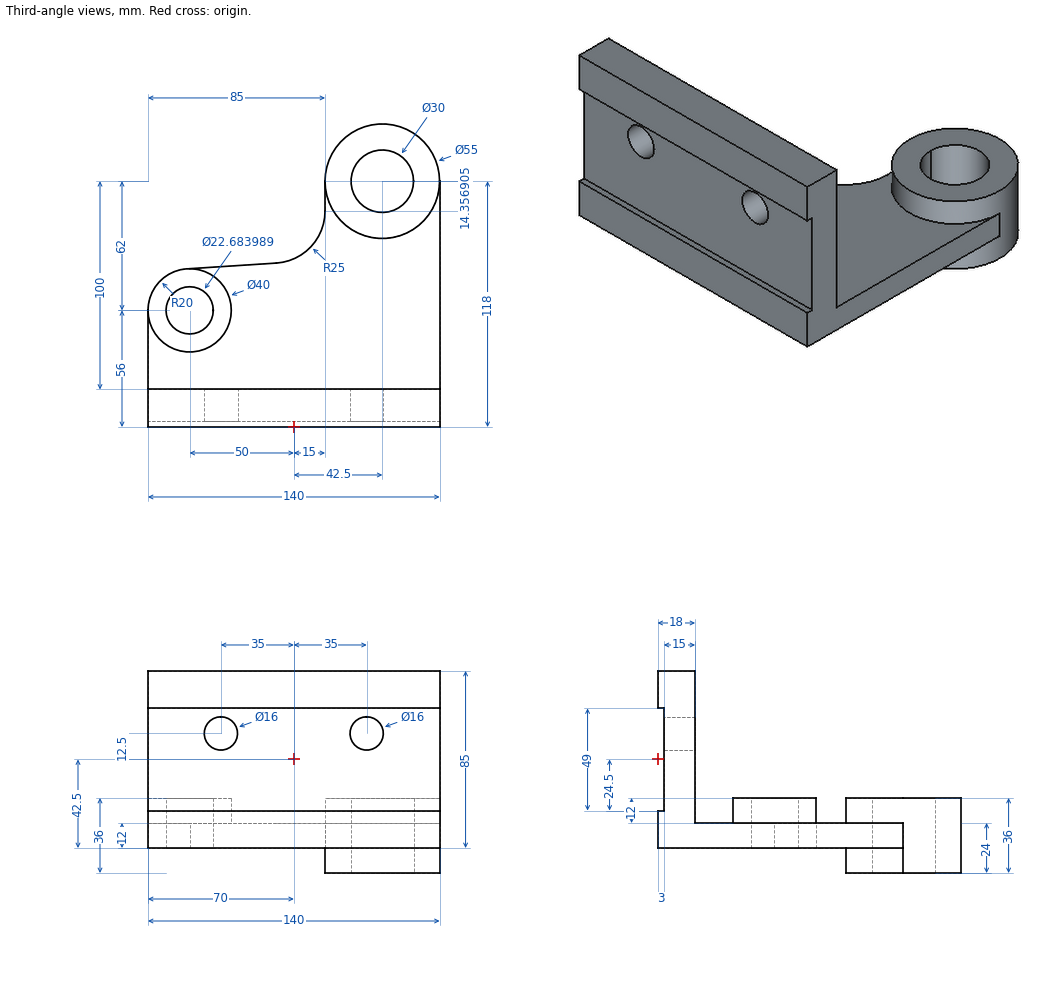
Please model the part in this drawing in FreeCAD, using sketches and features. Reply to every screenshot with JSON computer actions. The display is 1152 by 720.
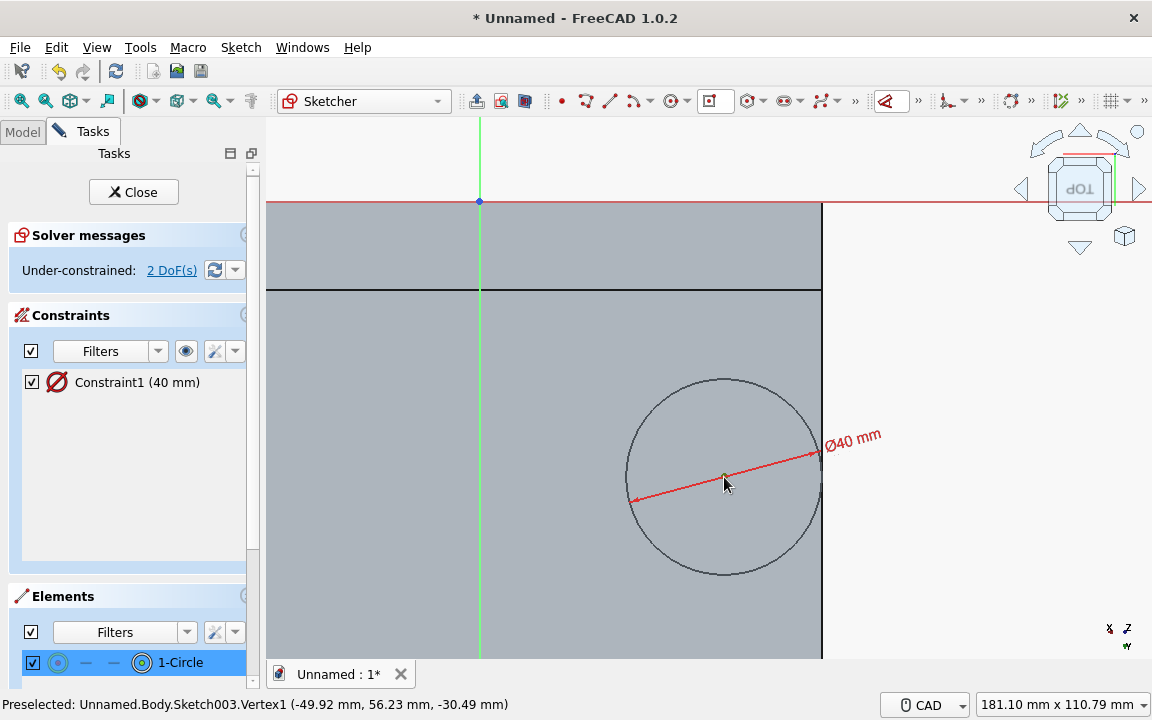
{"action": "key", "text": "l"}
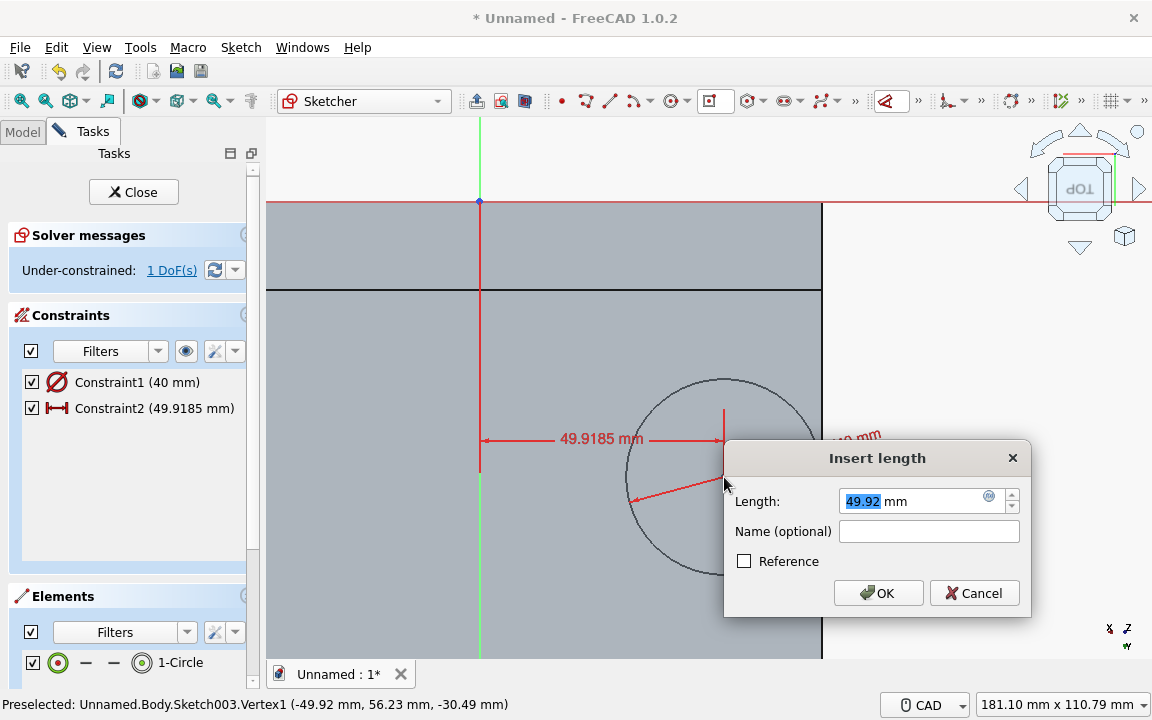
{"action": "type", "text": "50"}
{"action": "key", "text": "Return"}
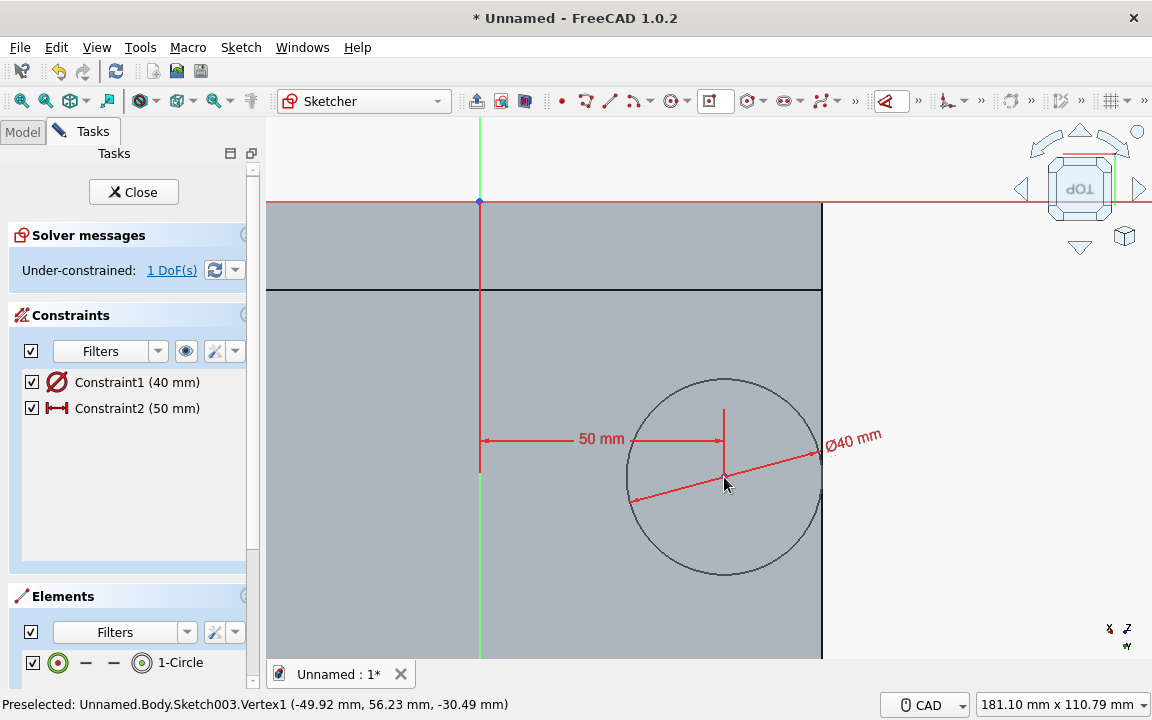
{"action": "left_click", "coordinate": [724, 477]}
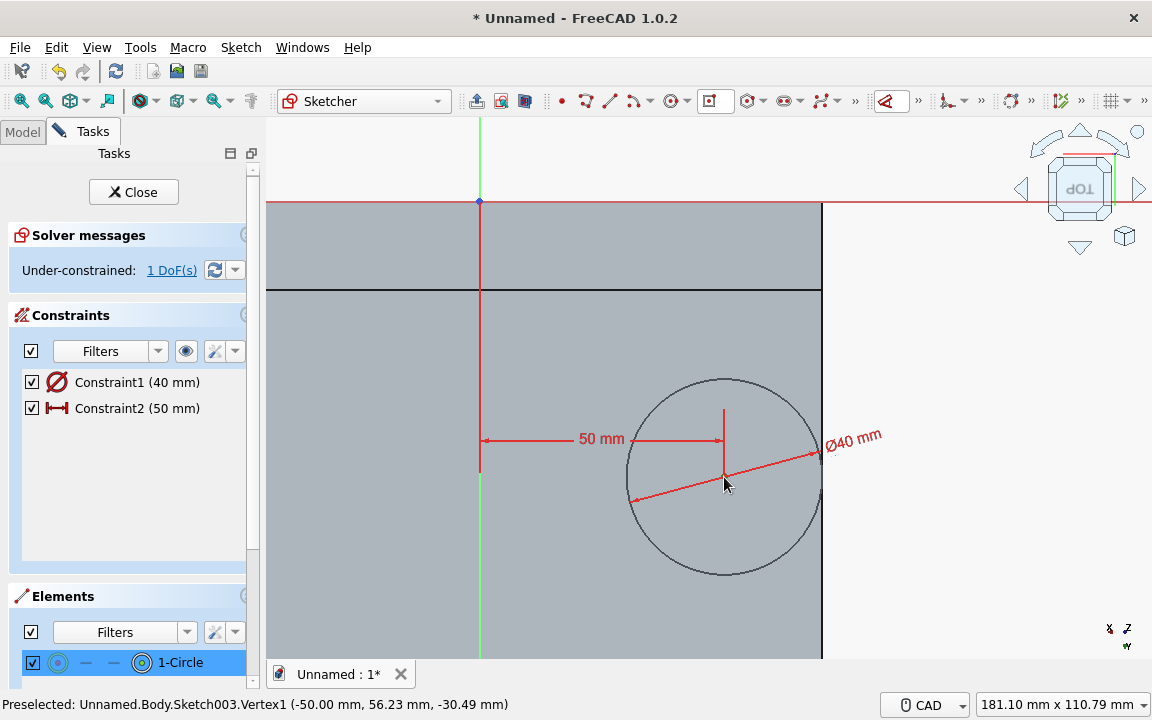
{"action": "key", "text": "i"}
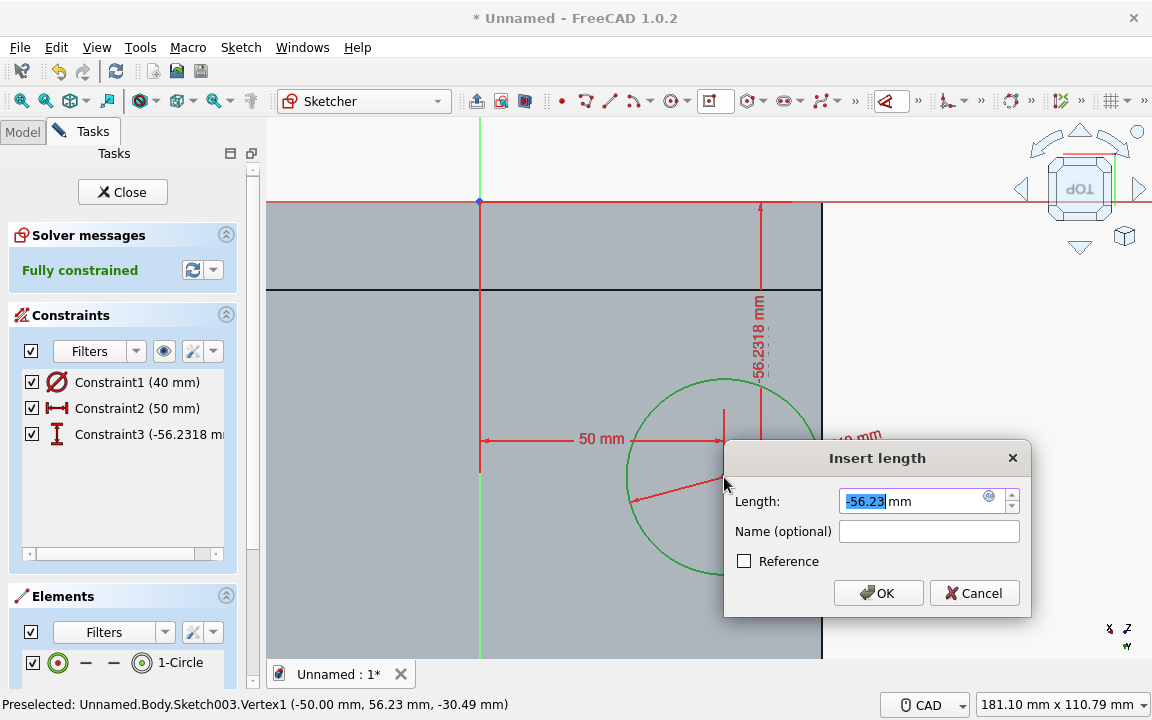
{"action": "type", "text": "-56"}
{"action": "key", "text": "Return"}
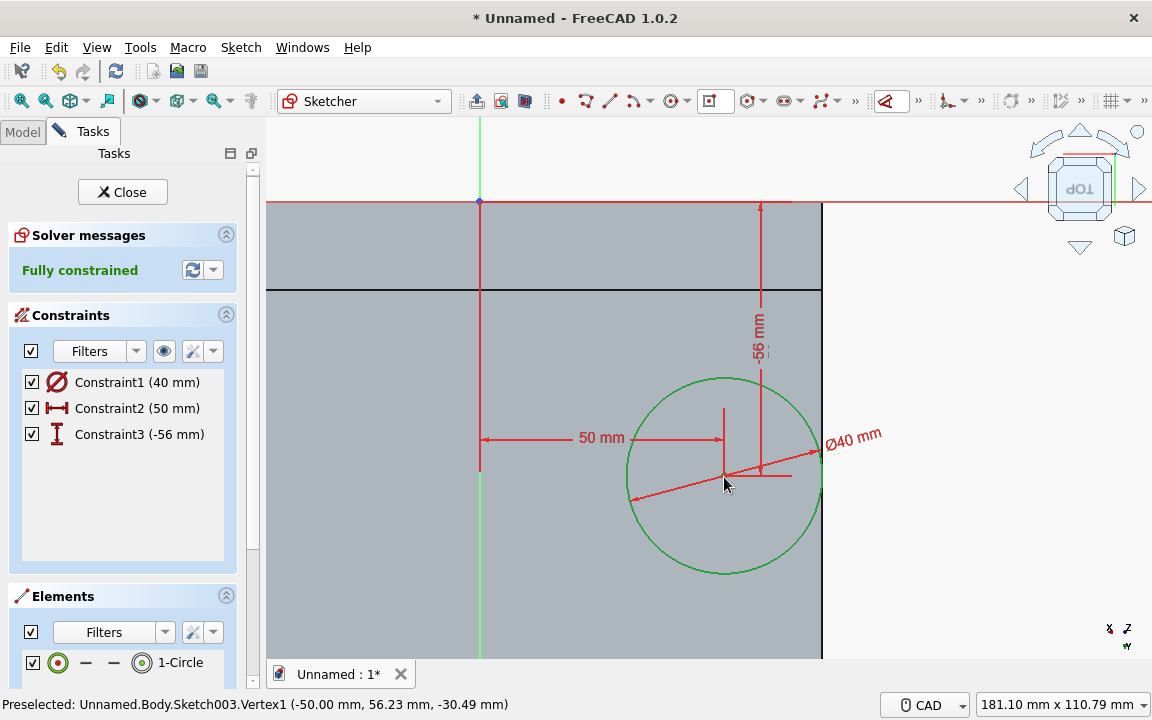
{"action": "left_click", "coordinate": [123, 192]}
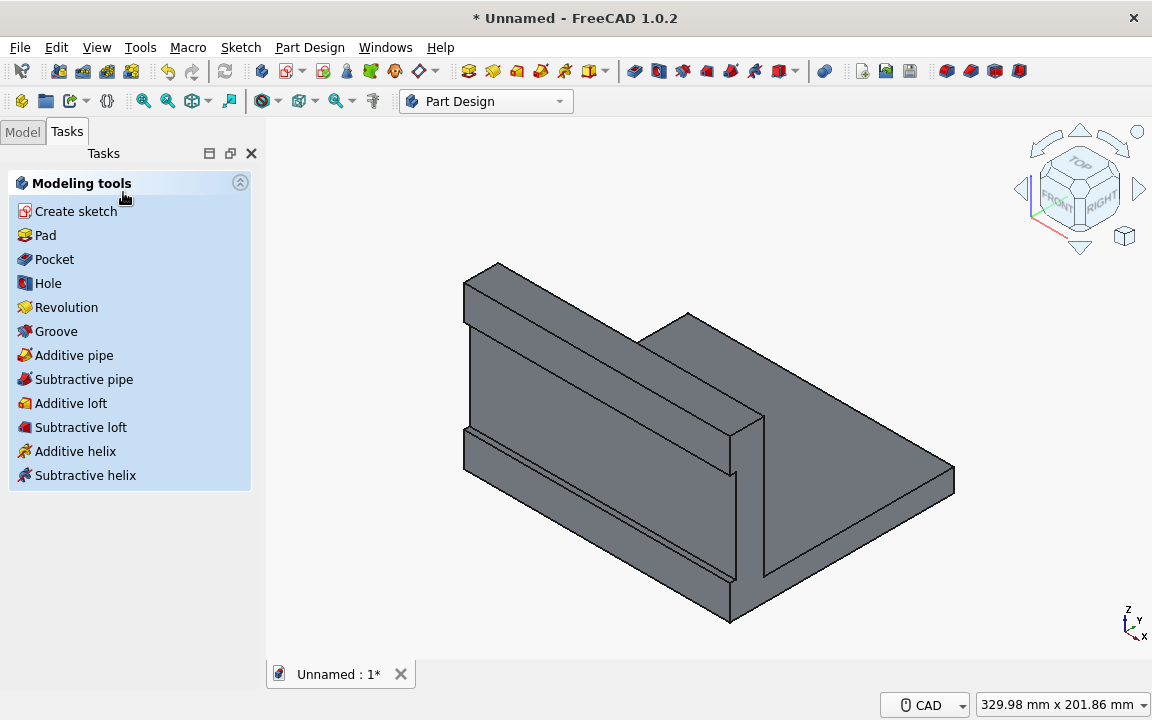
{"action": "left_click", "coordinate": [470, 72]}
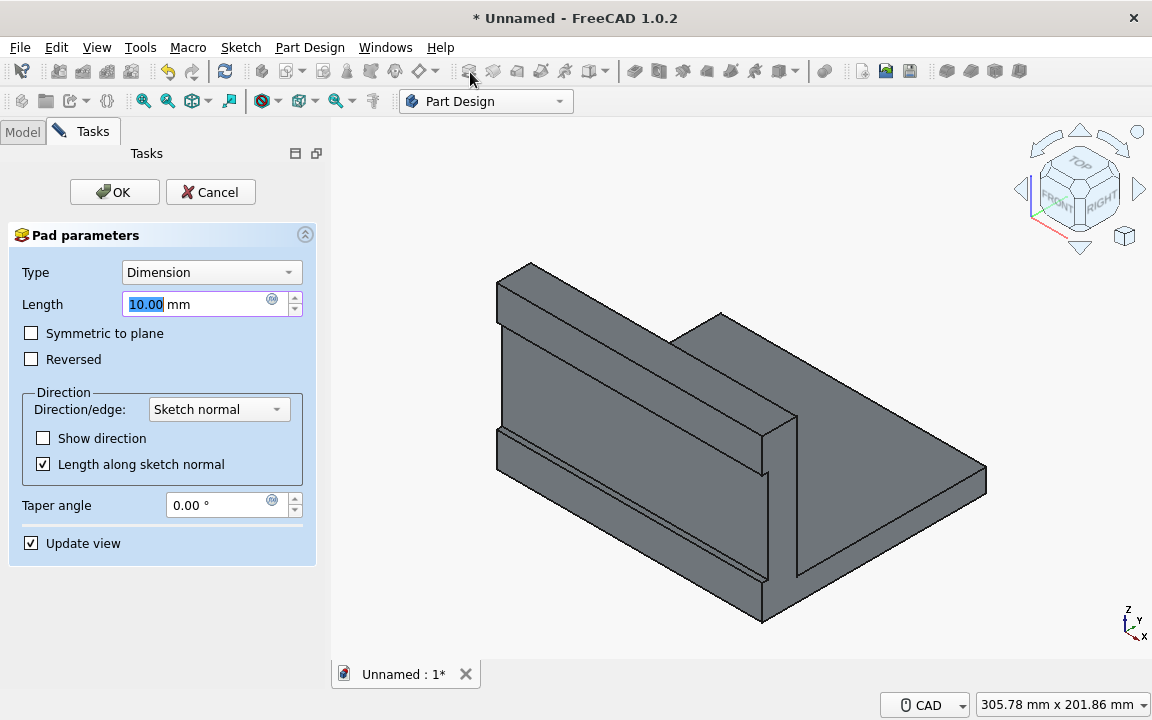
{"action": "type", "text": "12"}
{"action": "key", "text": "Tab"}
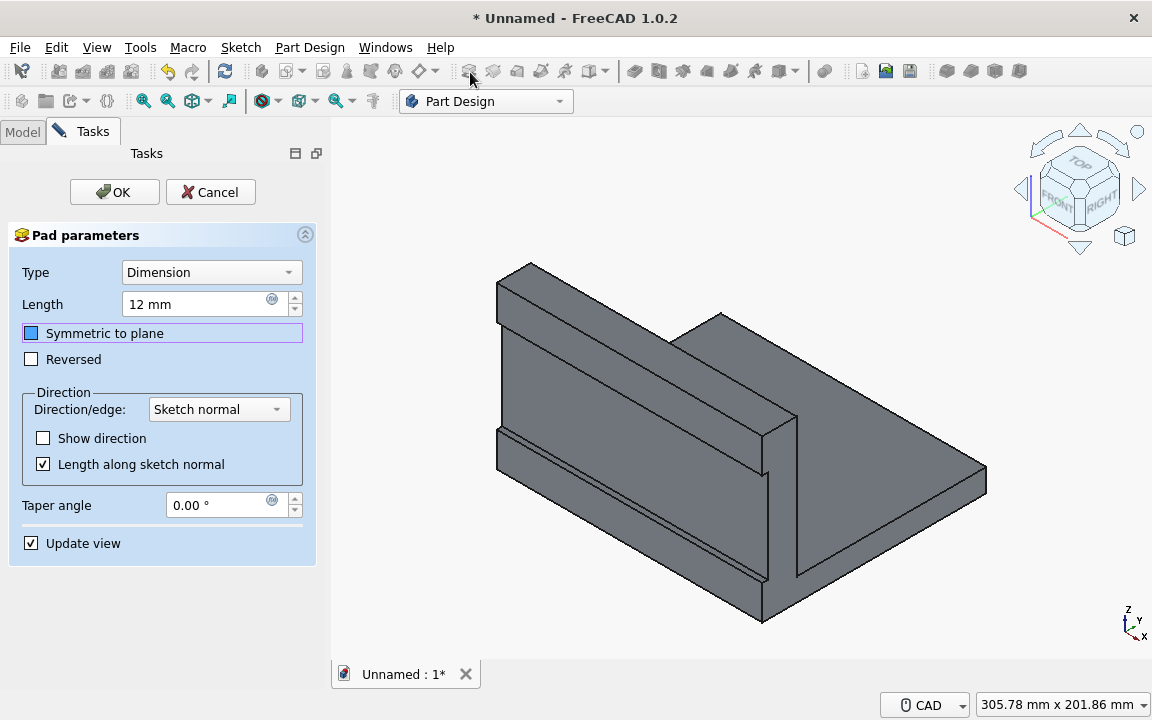
{"action": "left_click", "coordinate": [115, 192]}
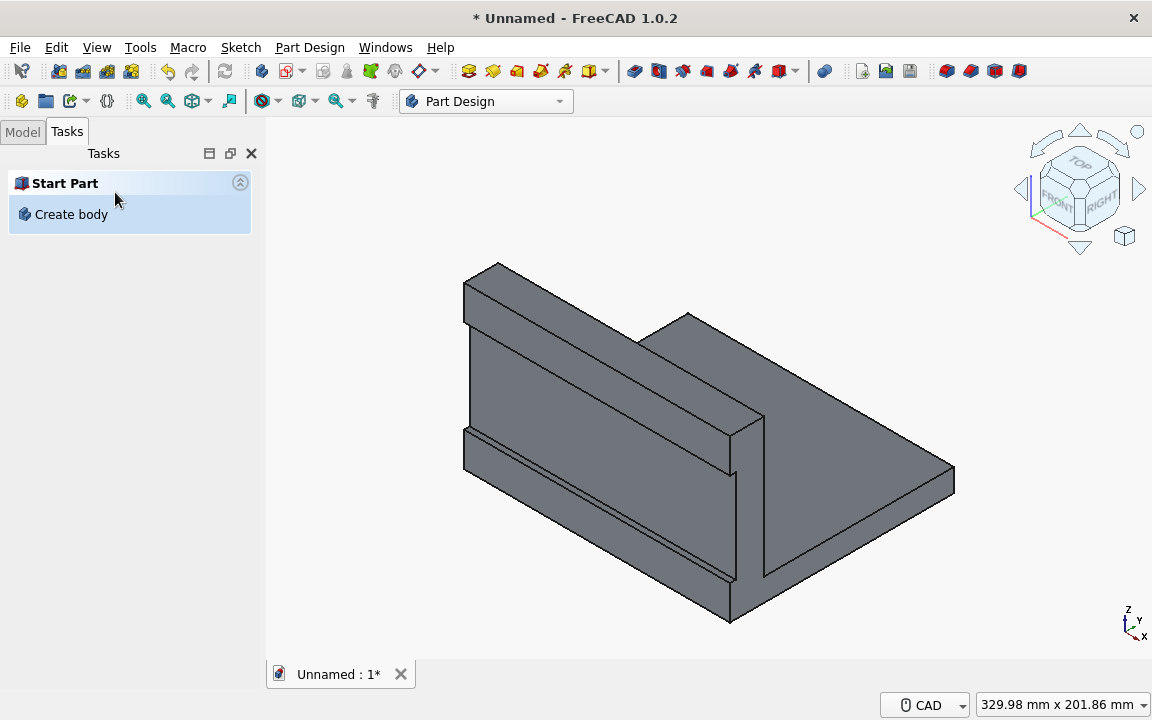
{"action": "left_click", "coordinate": [791, 450]}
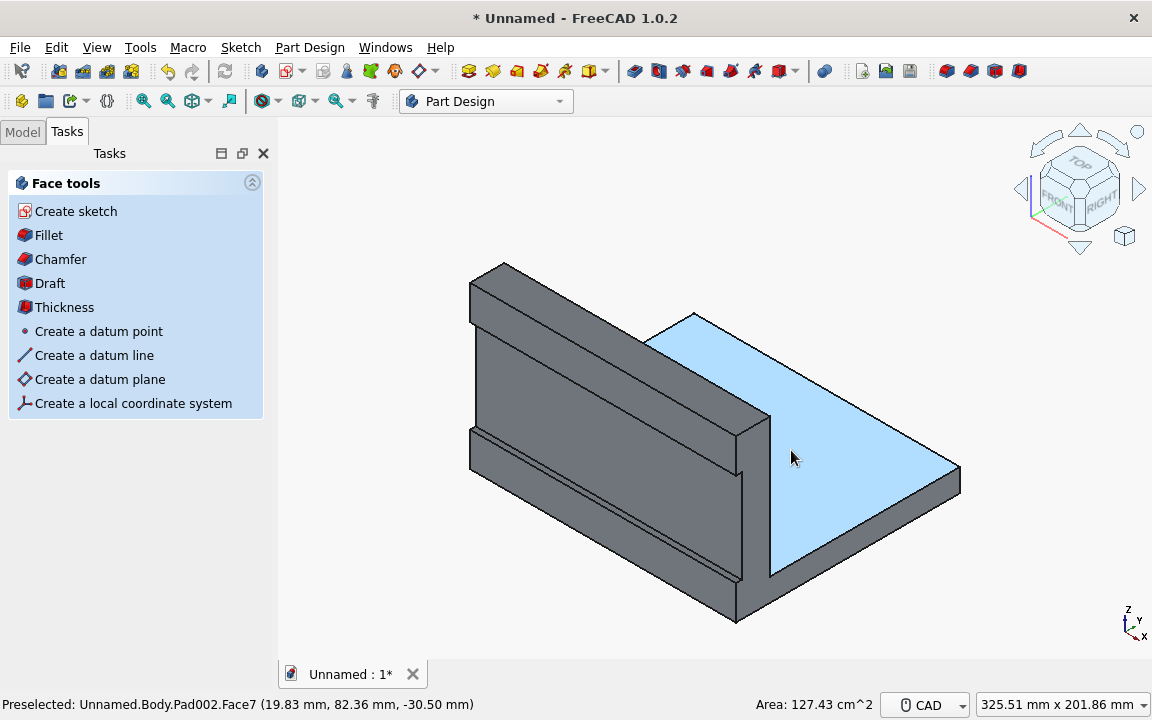
{"action": "left_click", "coordinate": [286, 72]}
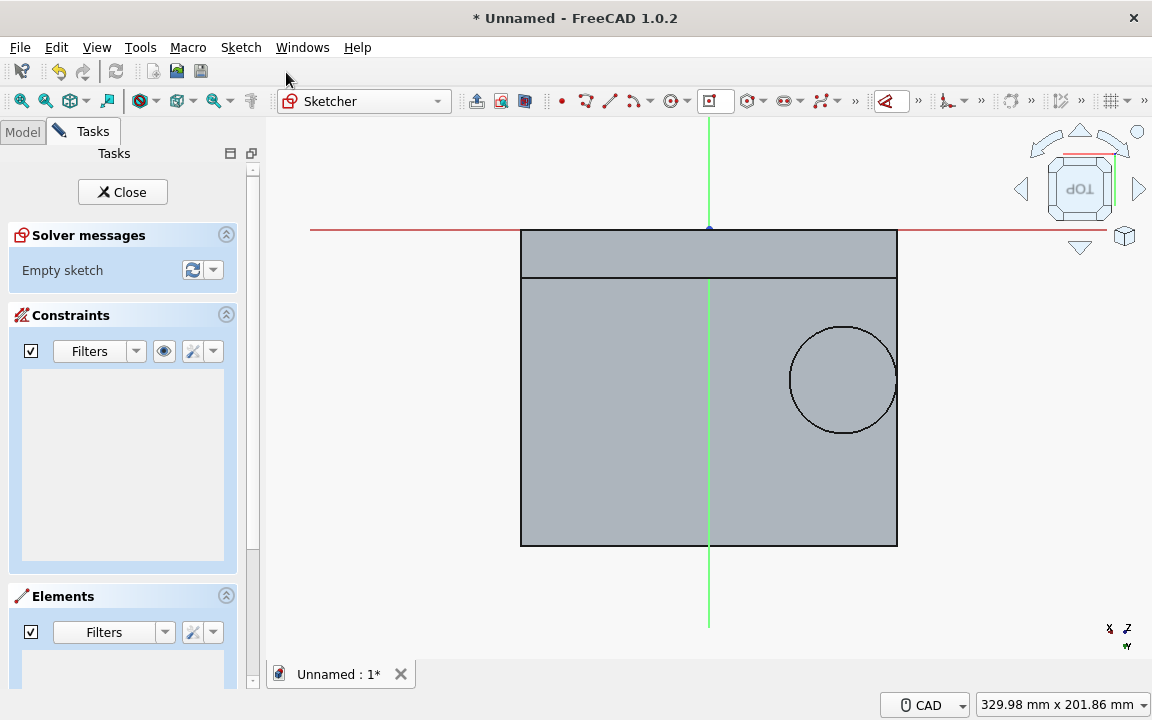
{"action": "scroll", "coordinate": [640, 388], "scroll_direction": "down", "scroll_amount": 5}